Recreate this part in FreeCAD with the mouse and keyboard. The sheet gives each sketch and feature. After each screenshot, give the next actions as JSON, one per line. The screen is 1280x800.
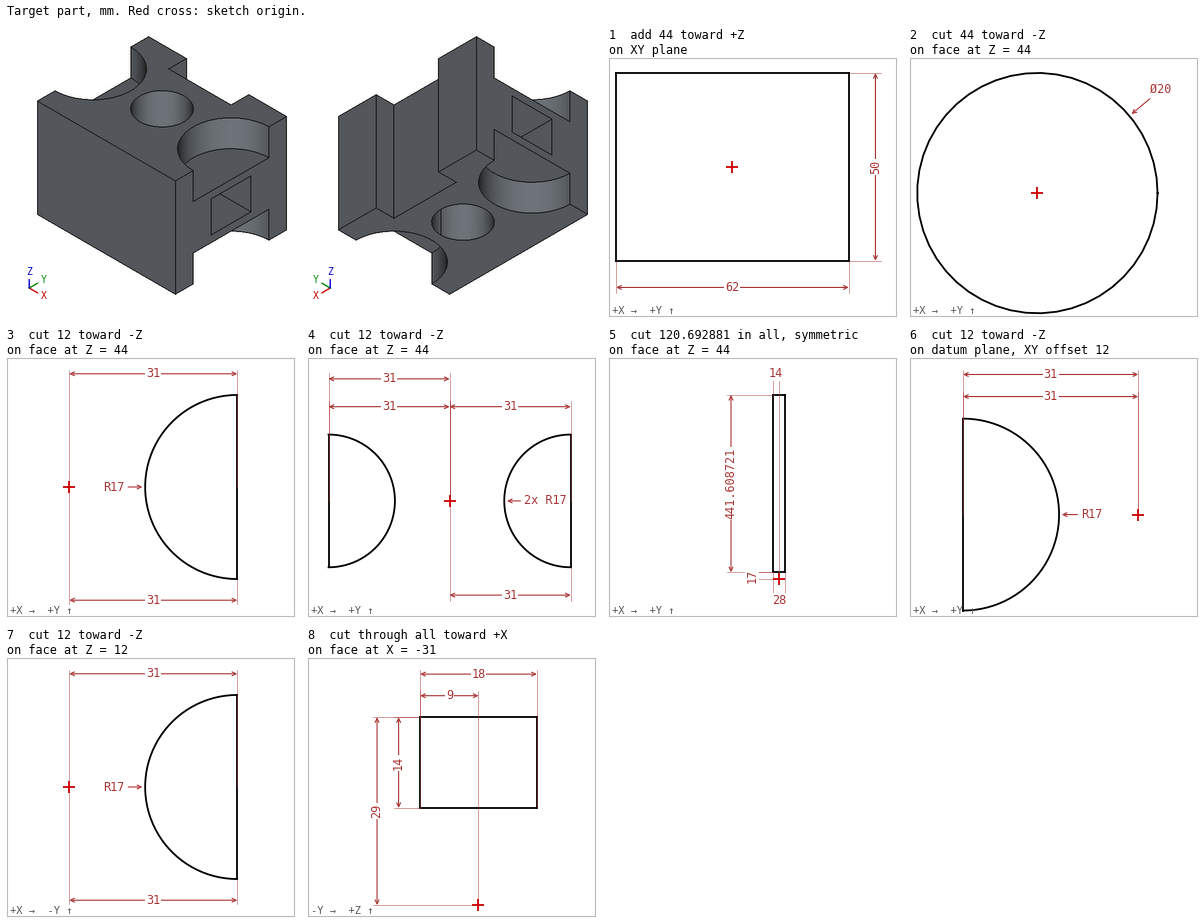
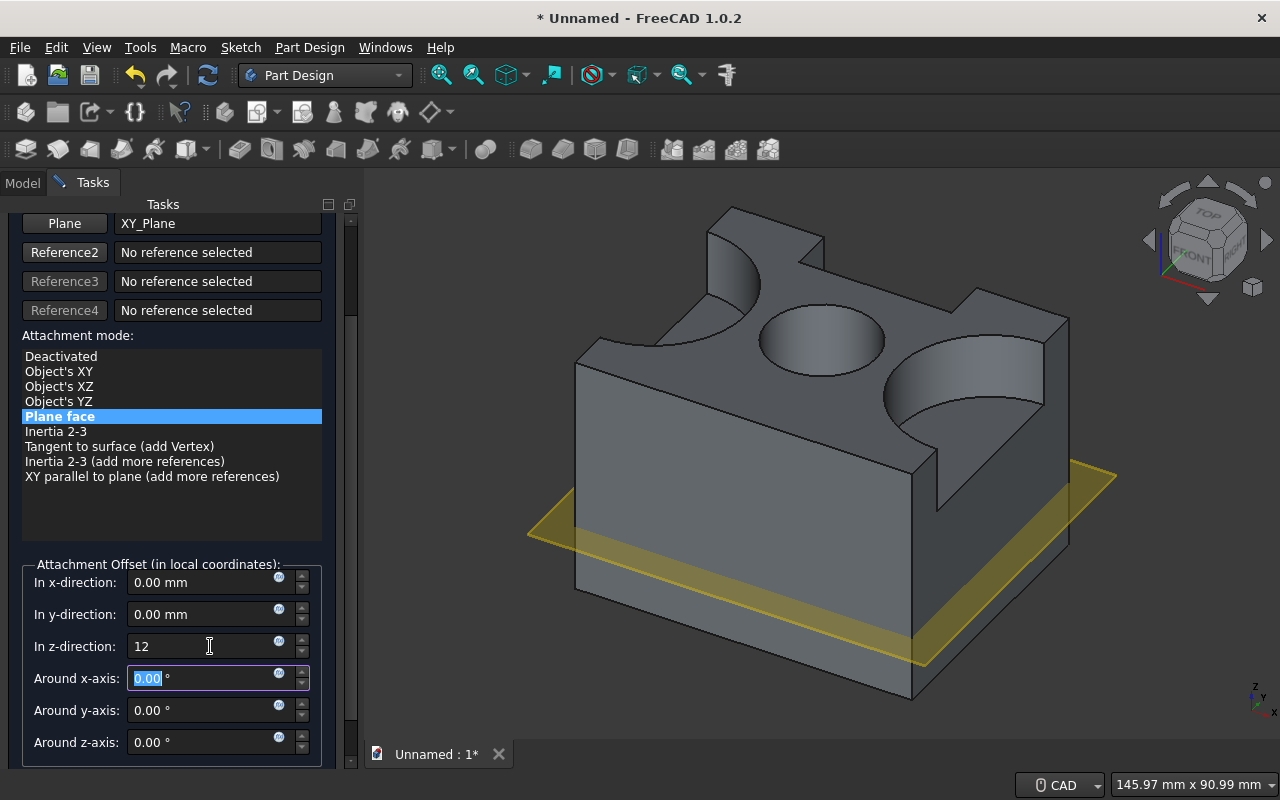
{"action": "scroll", "coordinate": [351, 491], "scroll_direction": "up", "scroll_amount": 3}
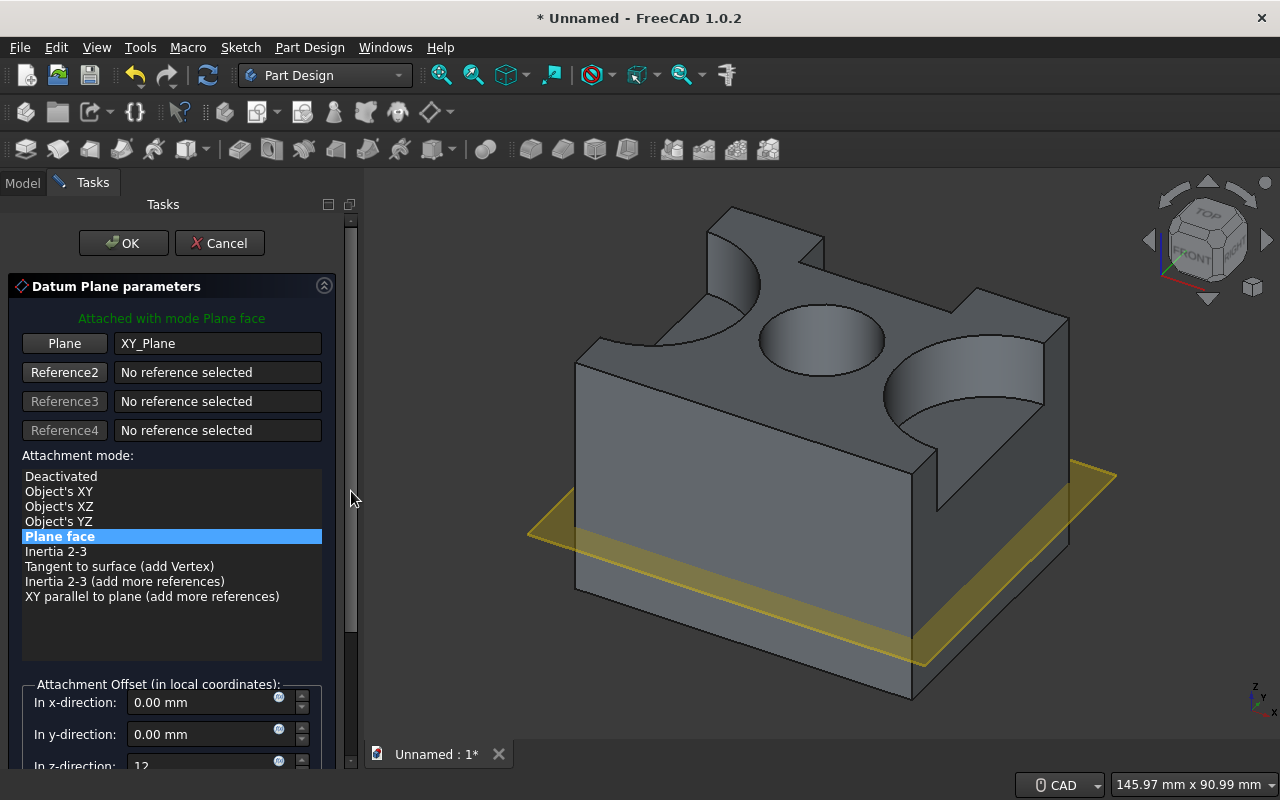
{"action": "left_click", "coordinate": [124, 243]}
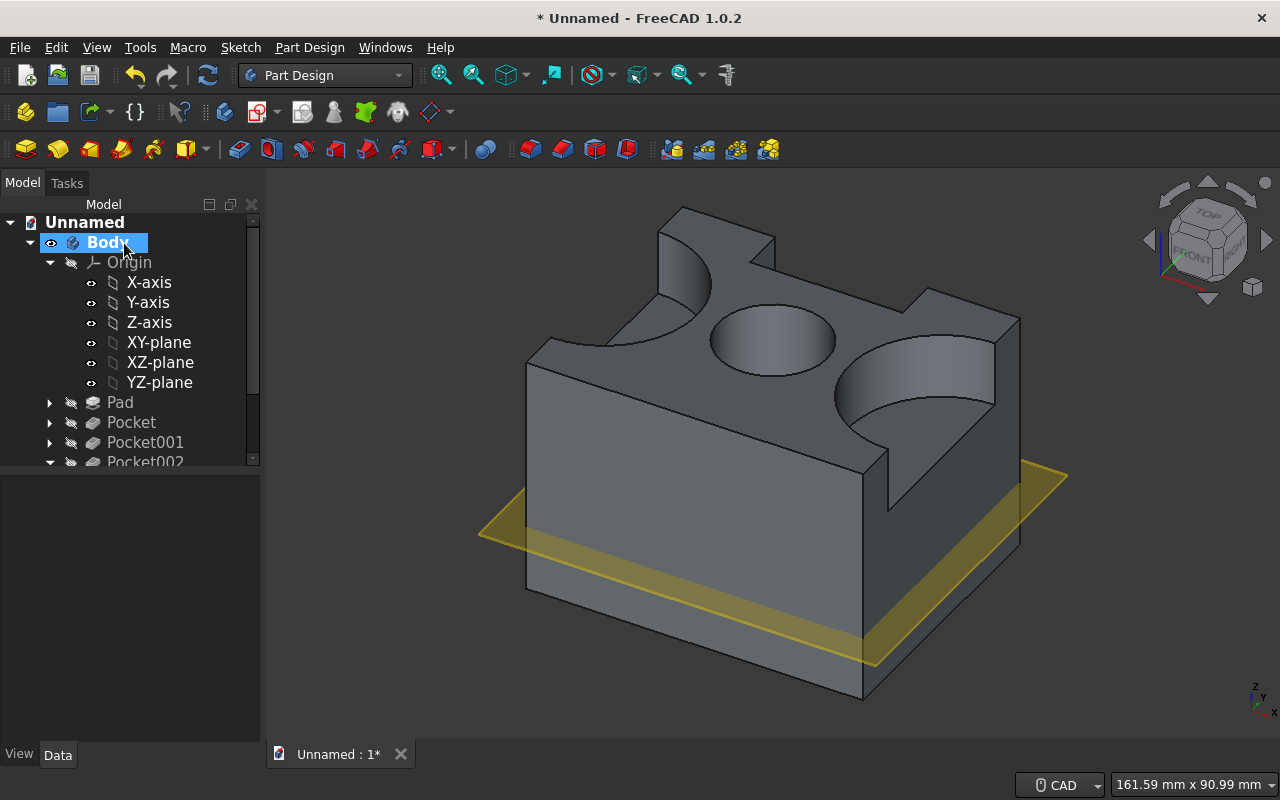
{"action": "scroll", "coordinate": [100, 338], "scroll_direction": "down", "scroll_amount": 3}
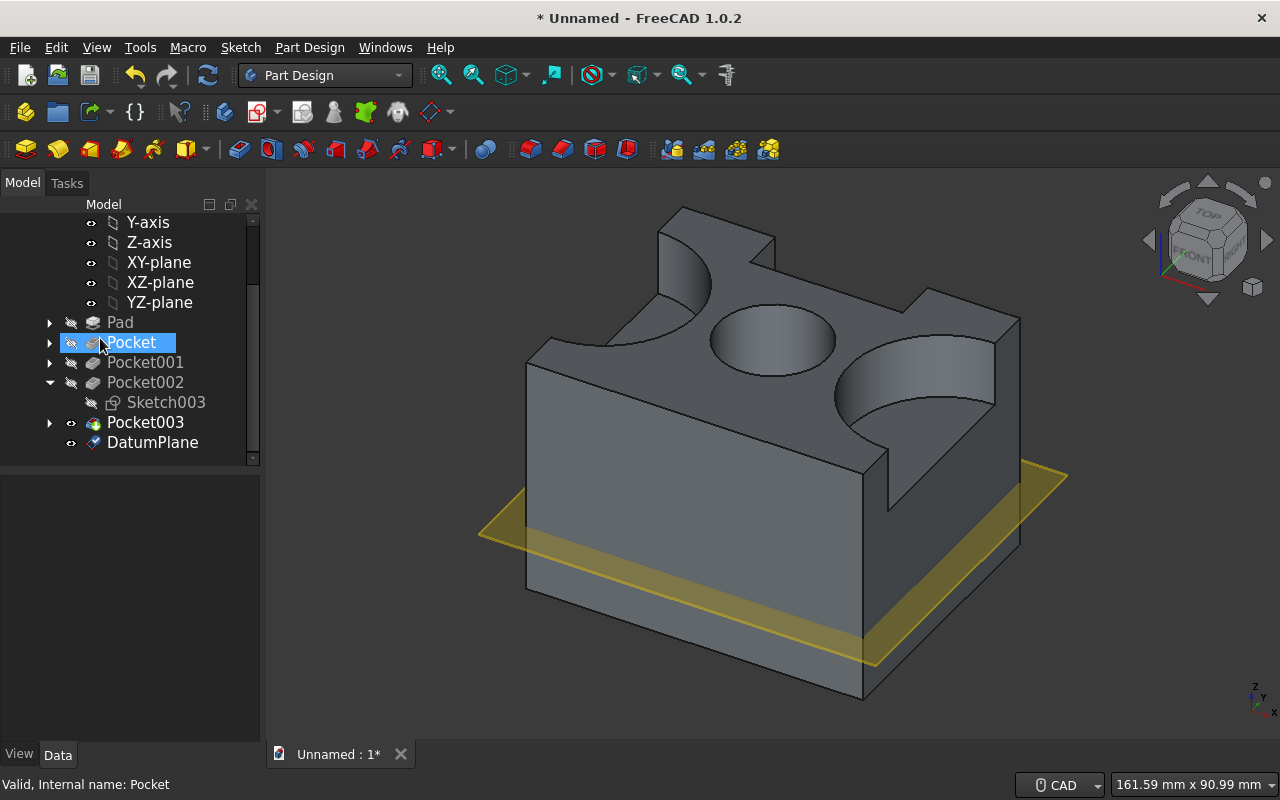
{"action": "left_click", "coordinate": [116, 443]}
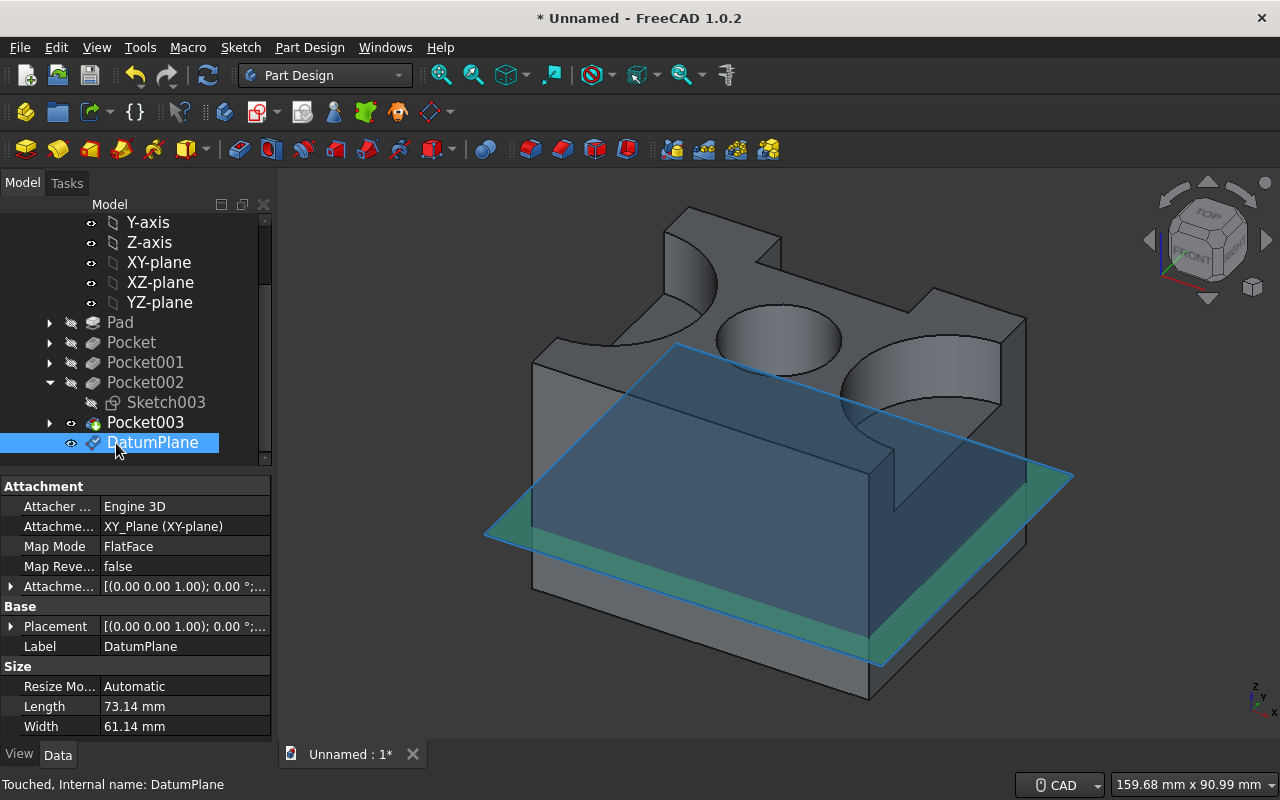
{"action": "left_click", "coordinate": [258, 112]}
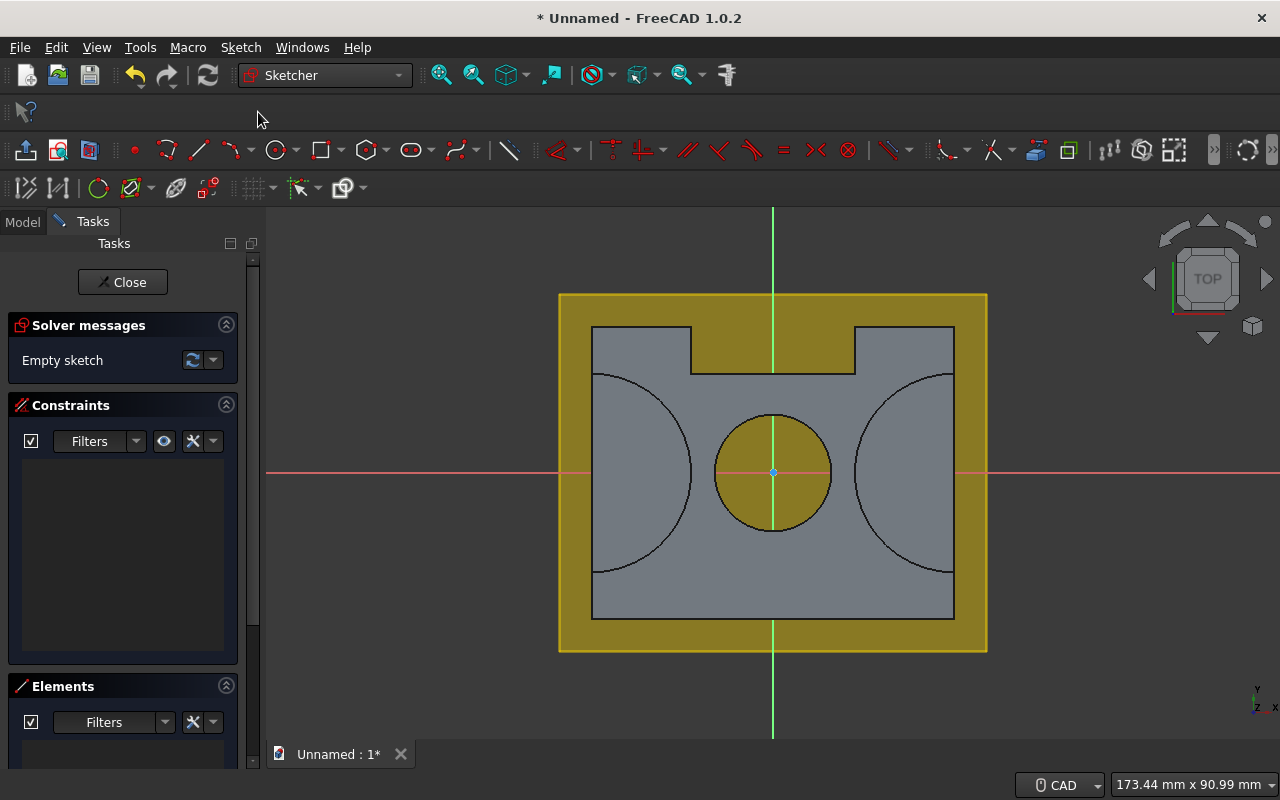
{"action": "left_click", "coordinate": [90, 150]}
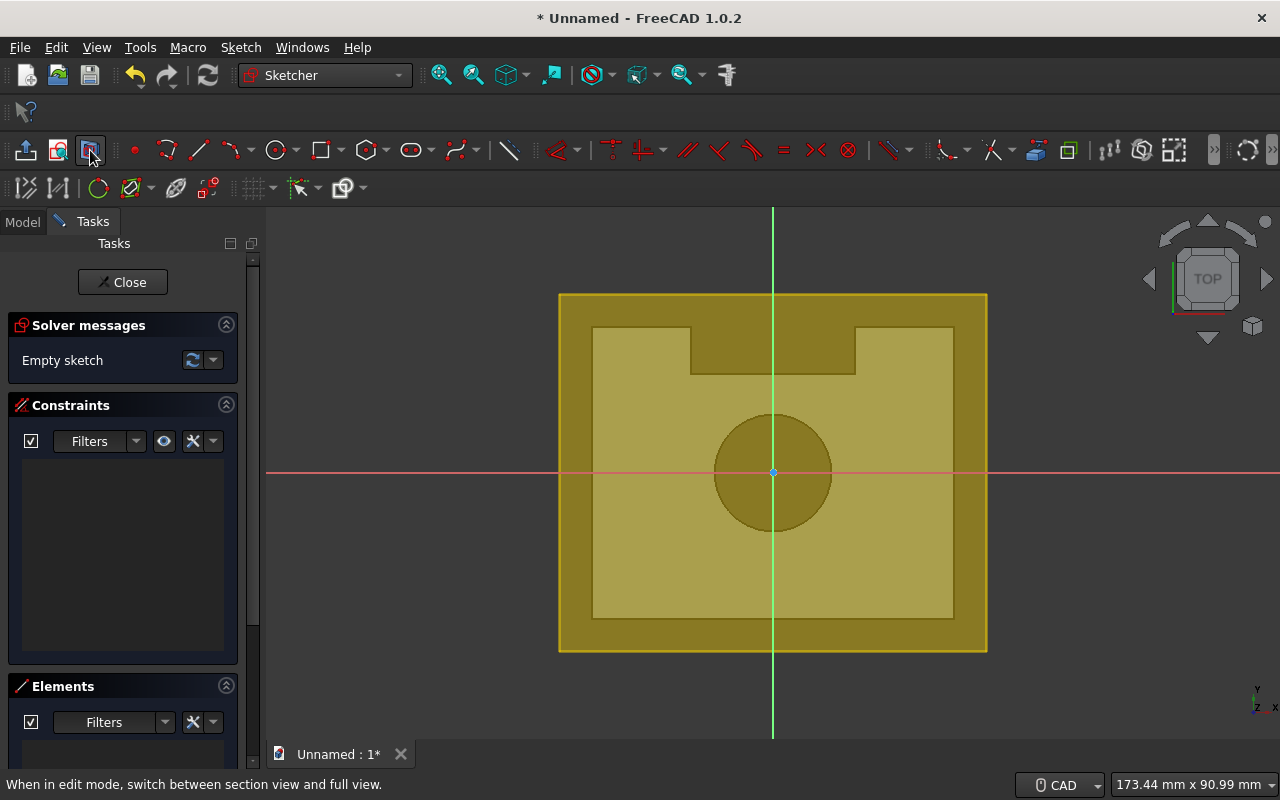
{"action": "scroll", "coordinate": [655, 473], "scroll_direction": "up", "scroll_amount": 3}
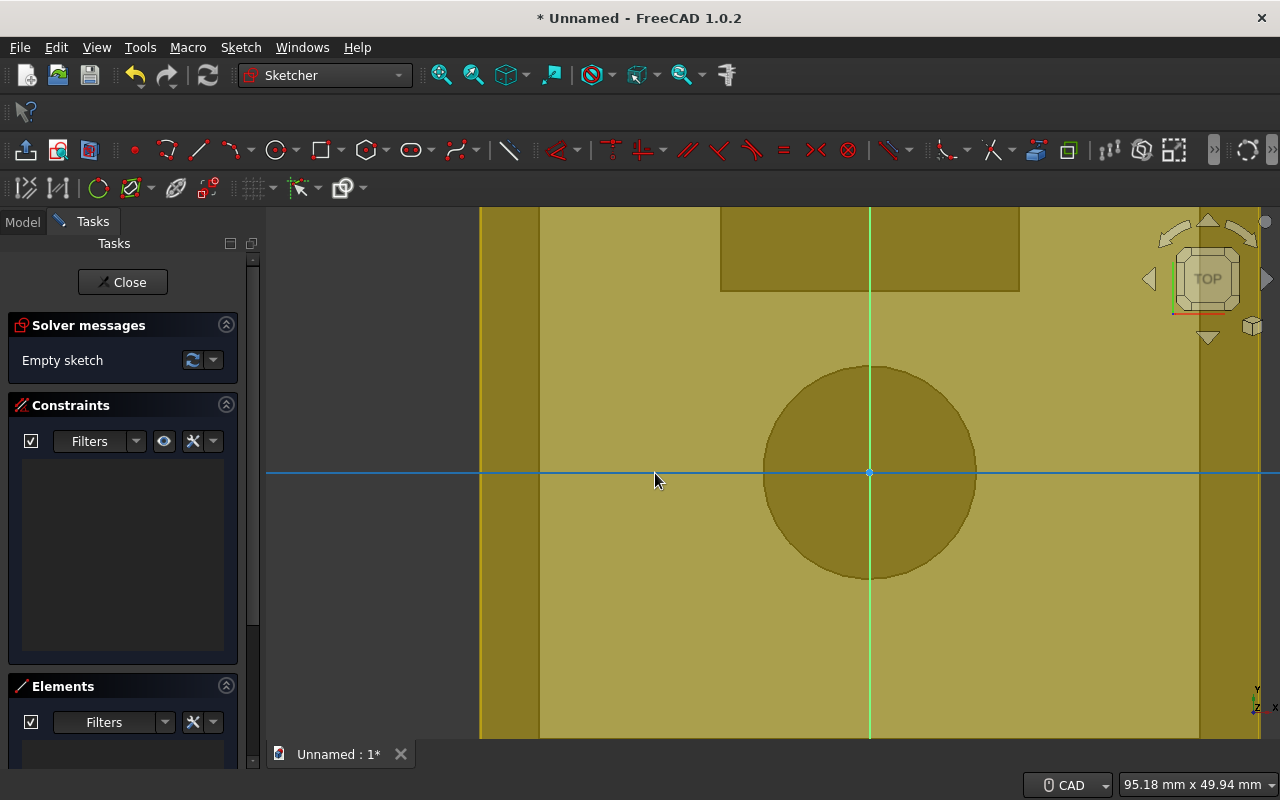
{"action": "key", "text": "g l"}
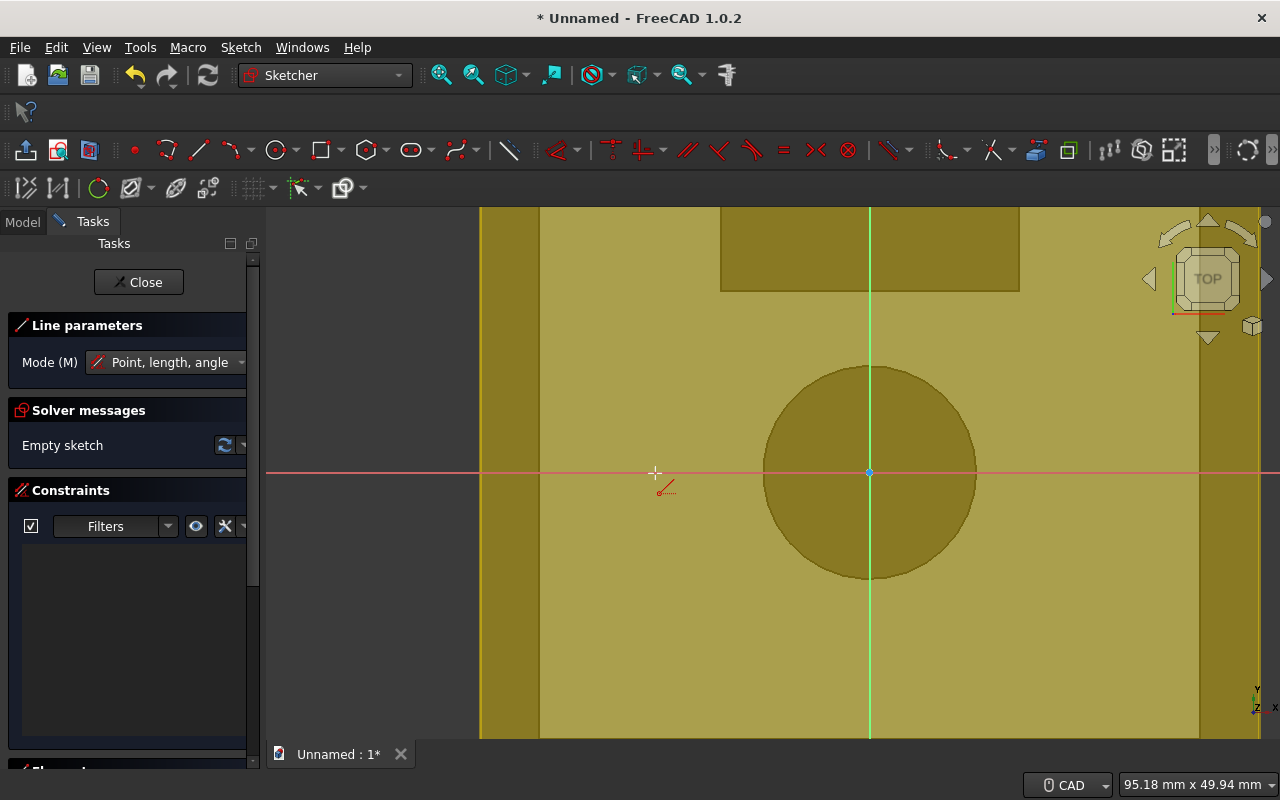
{"action": "left_click", "coordinate": [539, 291]}
{"action": "left_click", "coordinate": [539, 654]}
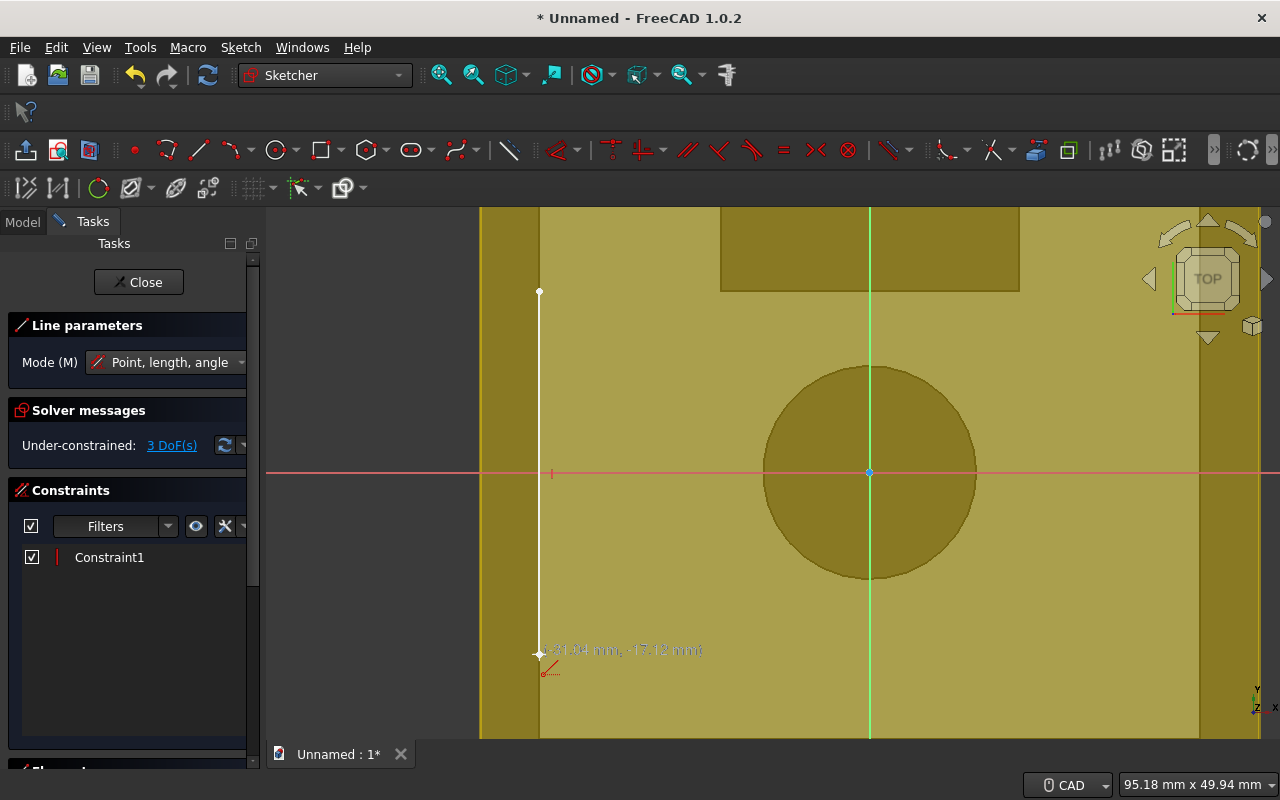
{"action": "key", "text": "g 3 a"}